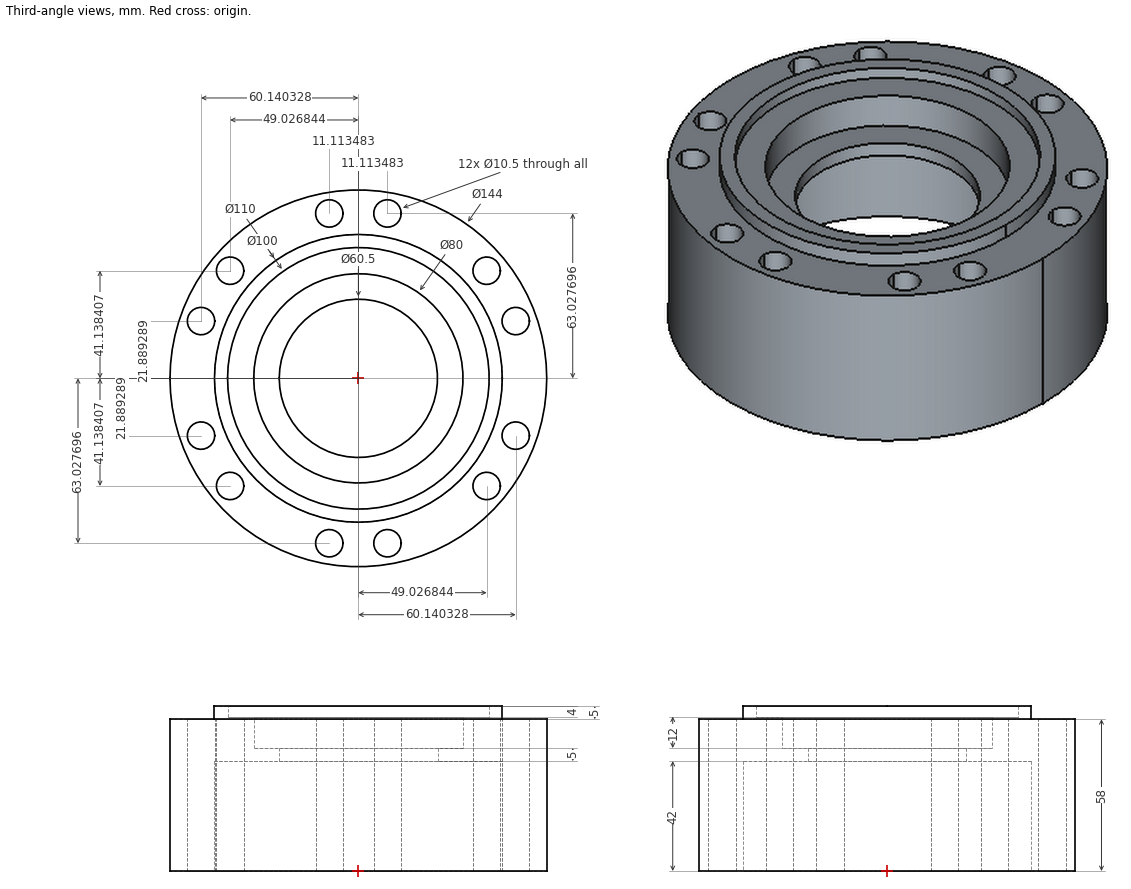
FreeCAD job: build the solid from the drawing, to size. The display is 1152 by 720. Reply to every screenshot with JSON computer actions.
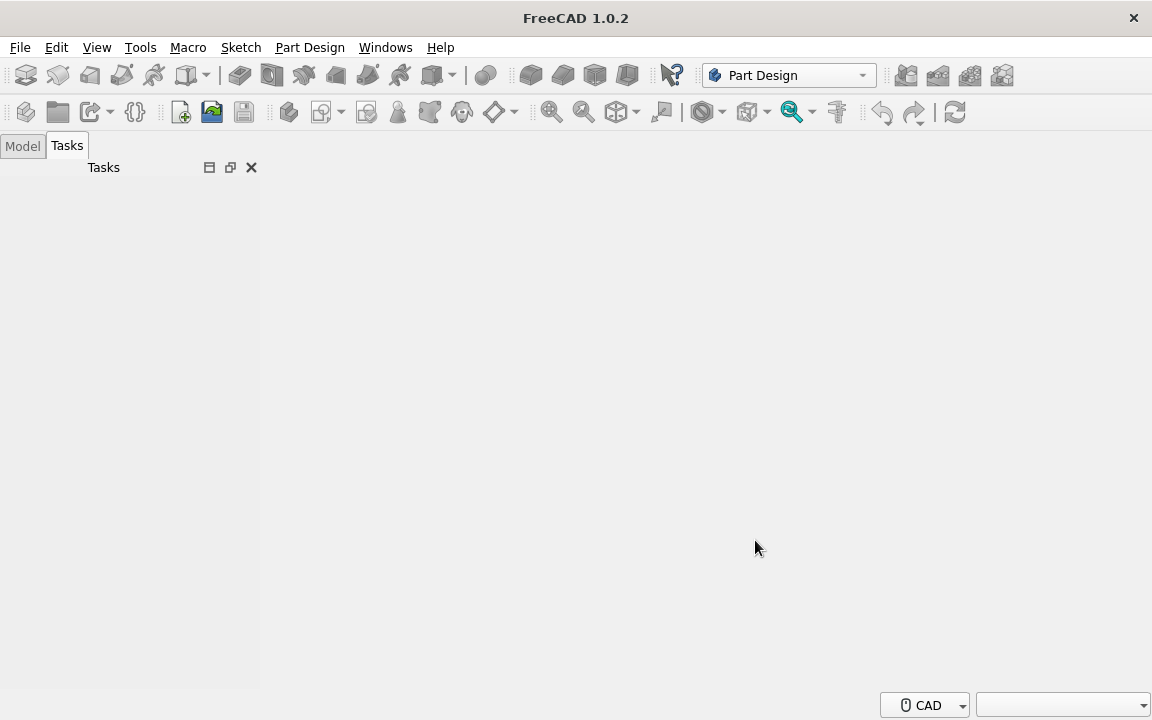
{"action": "left_click", "coordinate": [180, 112]}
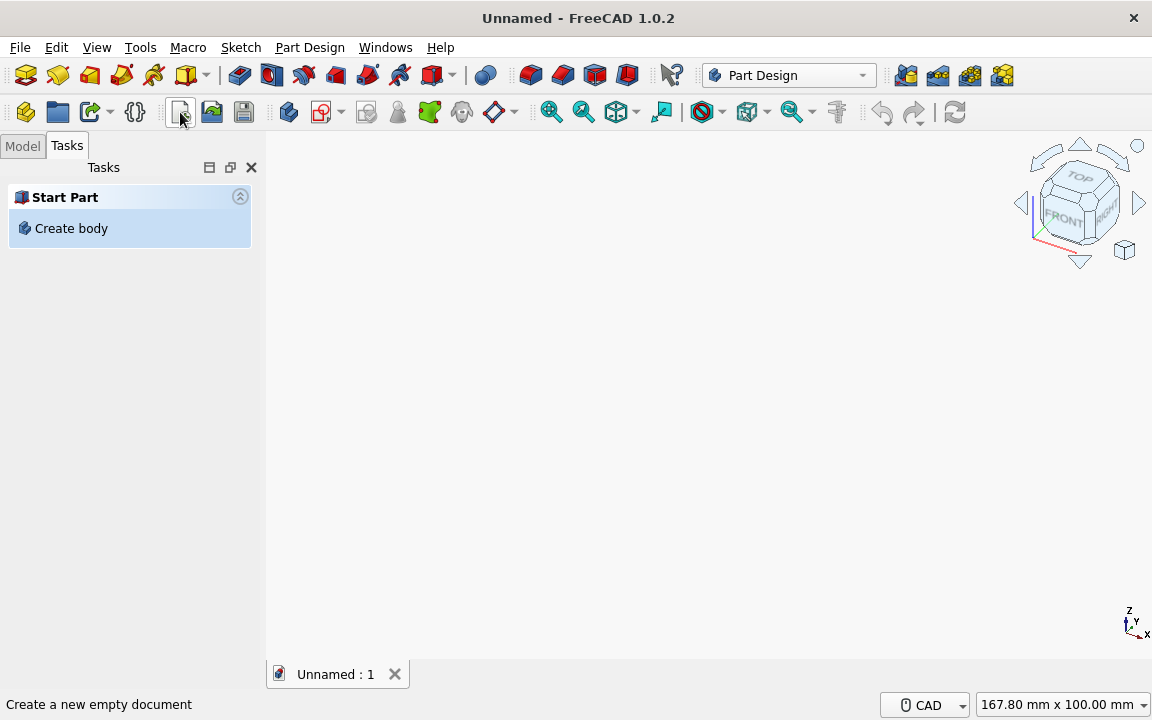
{"action": "left_click", "coordinate": [322, 112]}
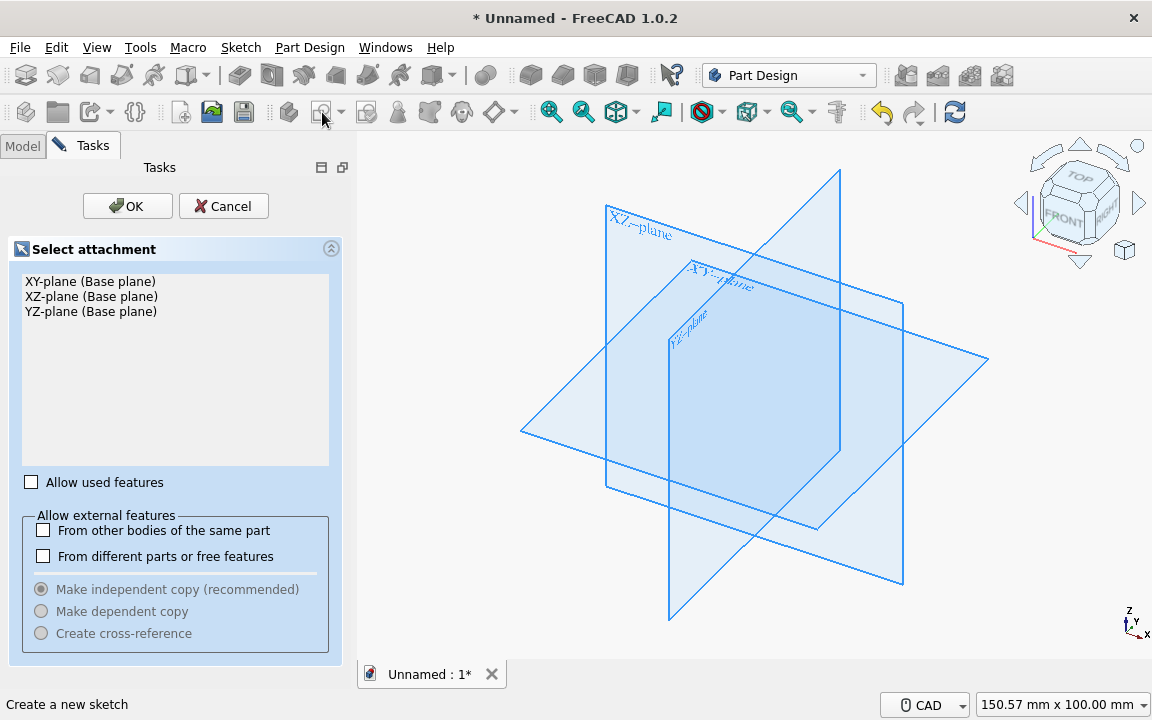
{"action": "left_click", "coordinate": [82, 282]}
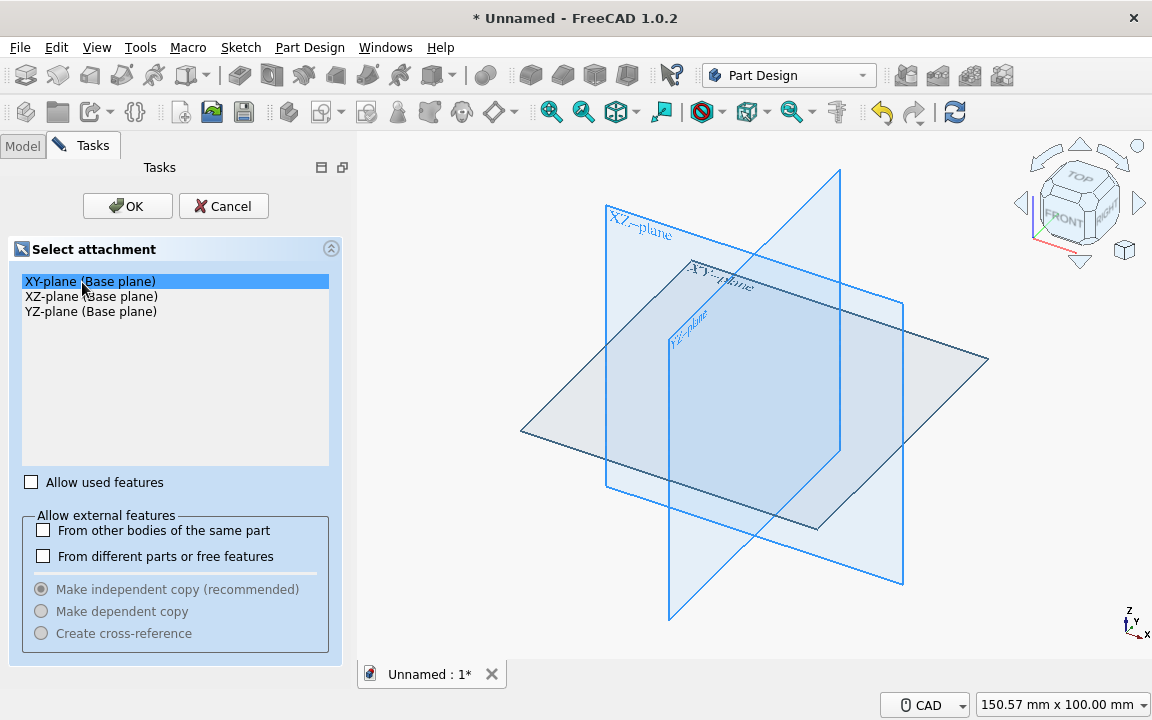
{"action": "left_click", "coordinate": [128, 206]}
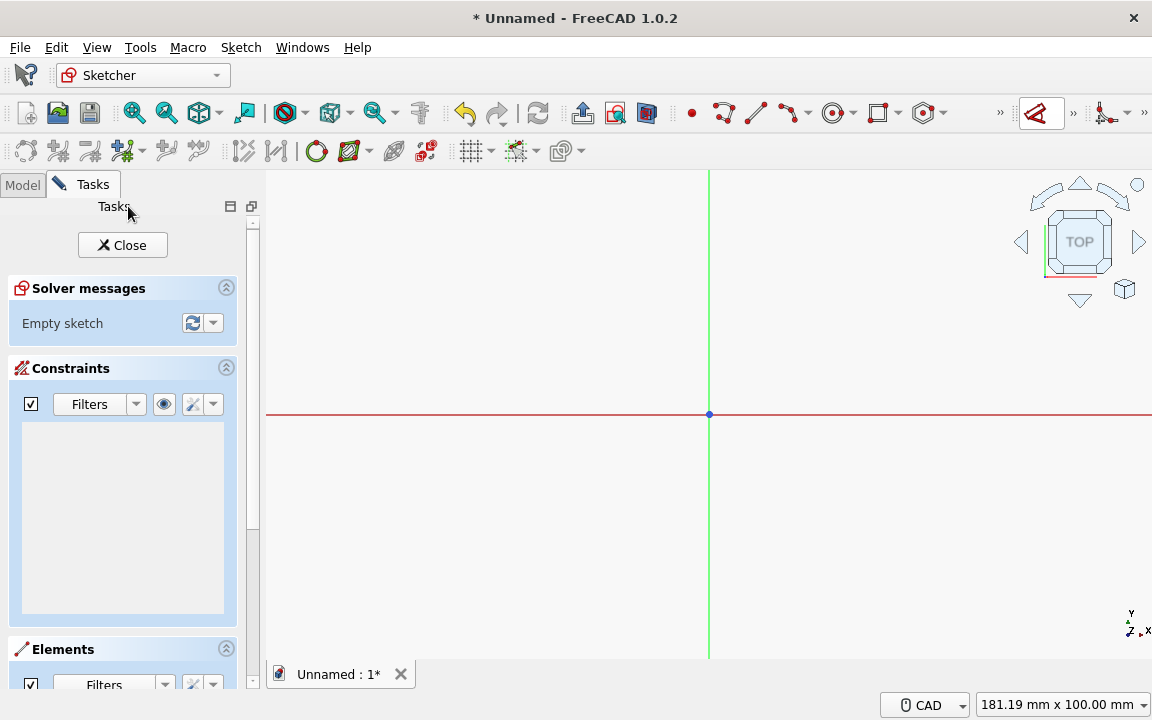
{"action": "scroll", "coordinate": [585, 414], "scroll_direction": "down", "scroll_amount": 4}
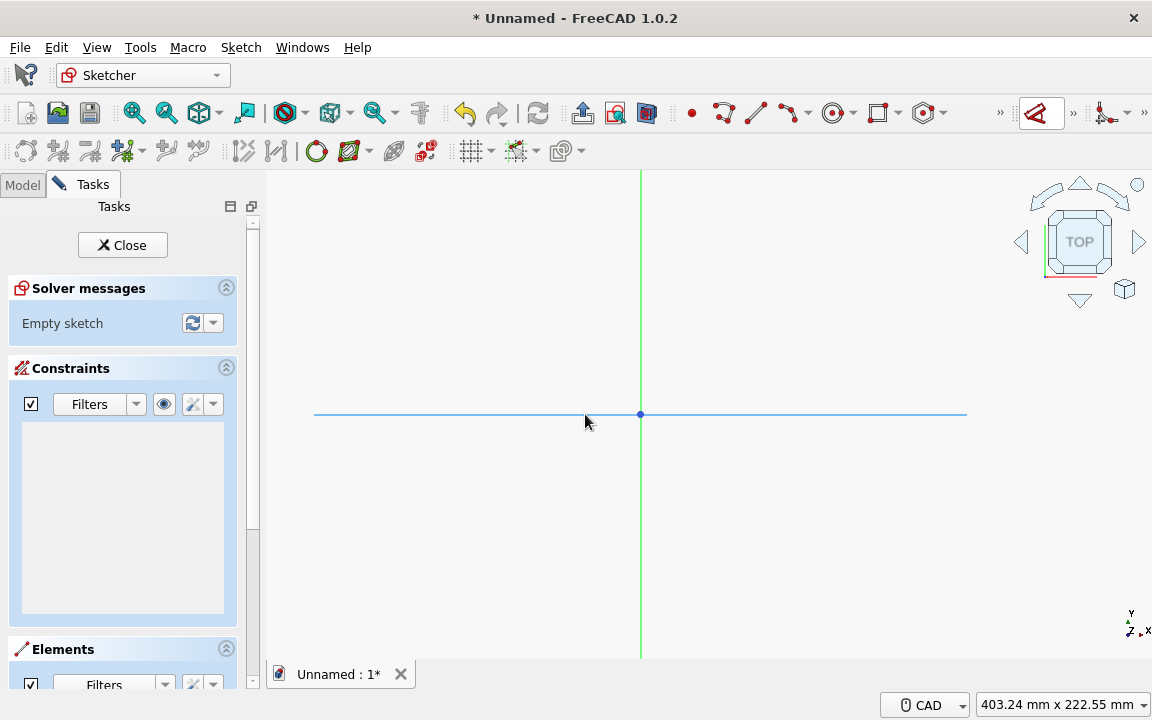
{"action": "left_click", "coordinate": [834, 114]}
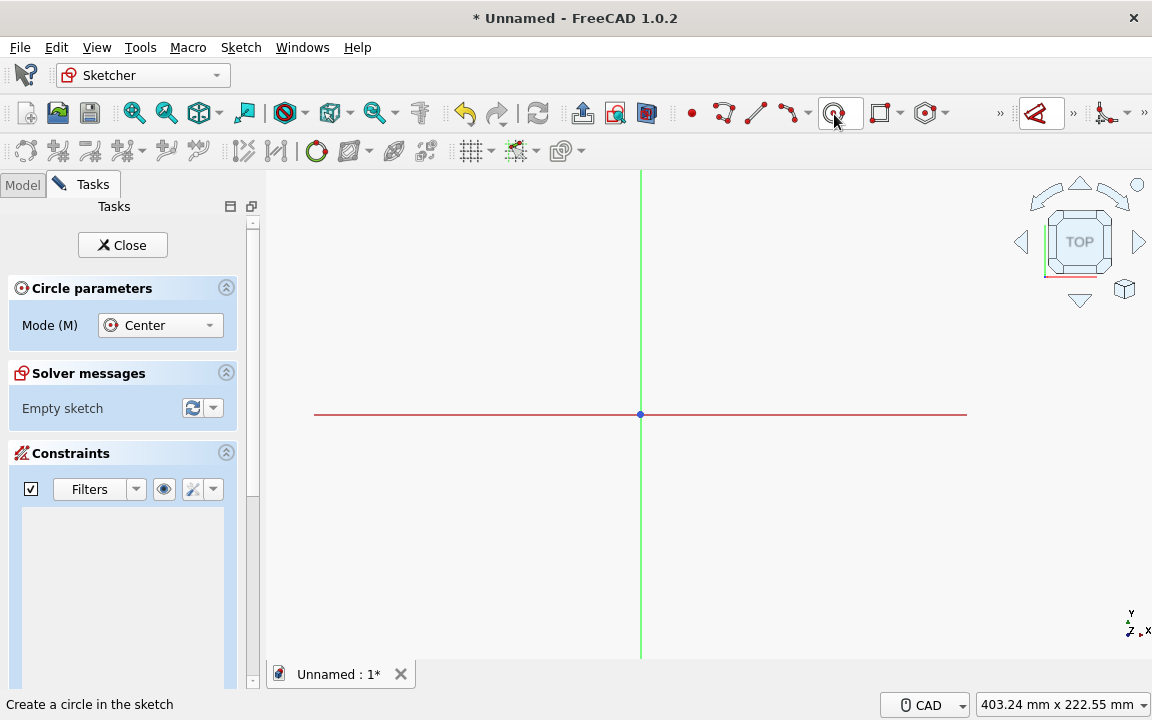
{"action": "left_click", "coordinate": [641, 414]}
{"action": "left_click", "coordinate": [753, 303]}
{"action": "key", "text": "Escape"}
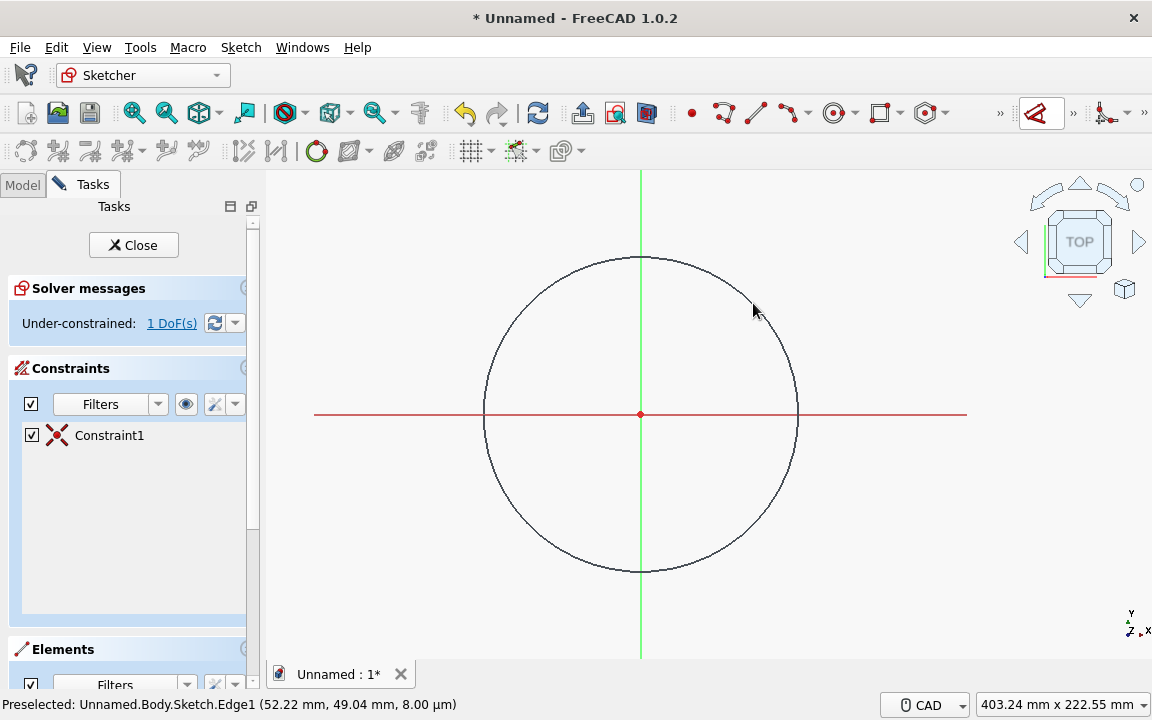
{"action": "key", "text": "d"}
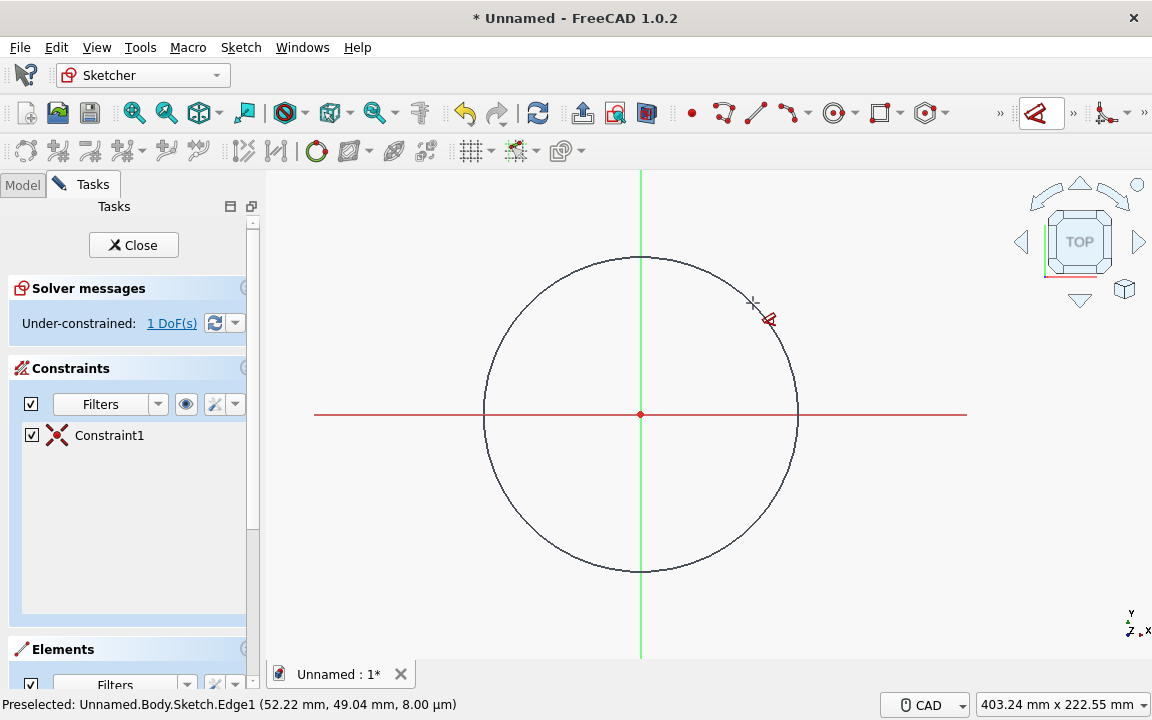
{"action": "left_click", "coordinate": [752, 303]}
{"action": "left_click", "coordinate": [775, 280]}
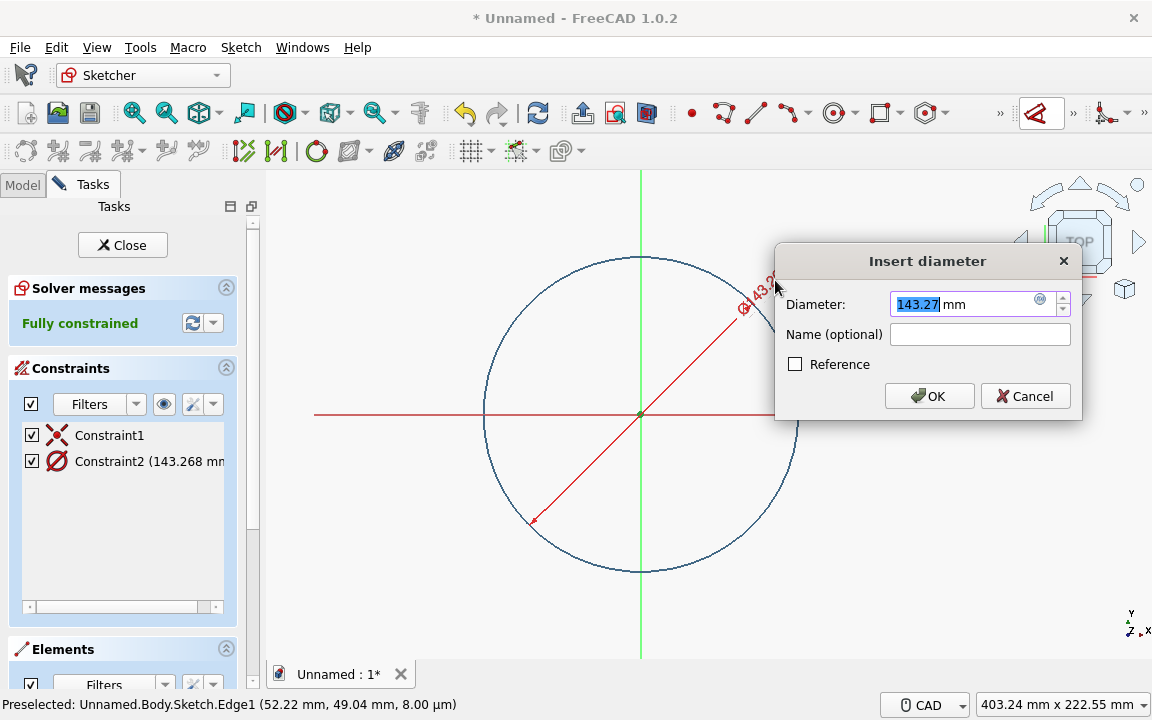
{"action": "type", "text": "144"}
{"action": "key", "text": "Return"}
{"action": "key", "text": "Escape"}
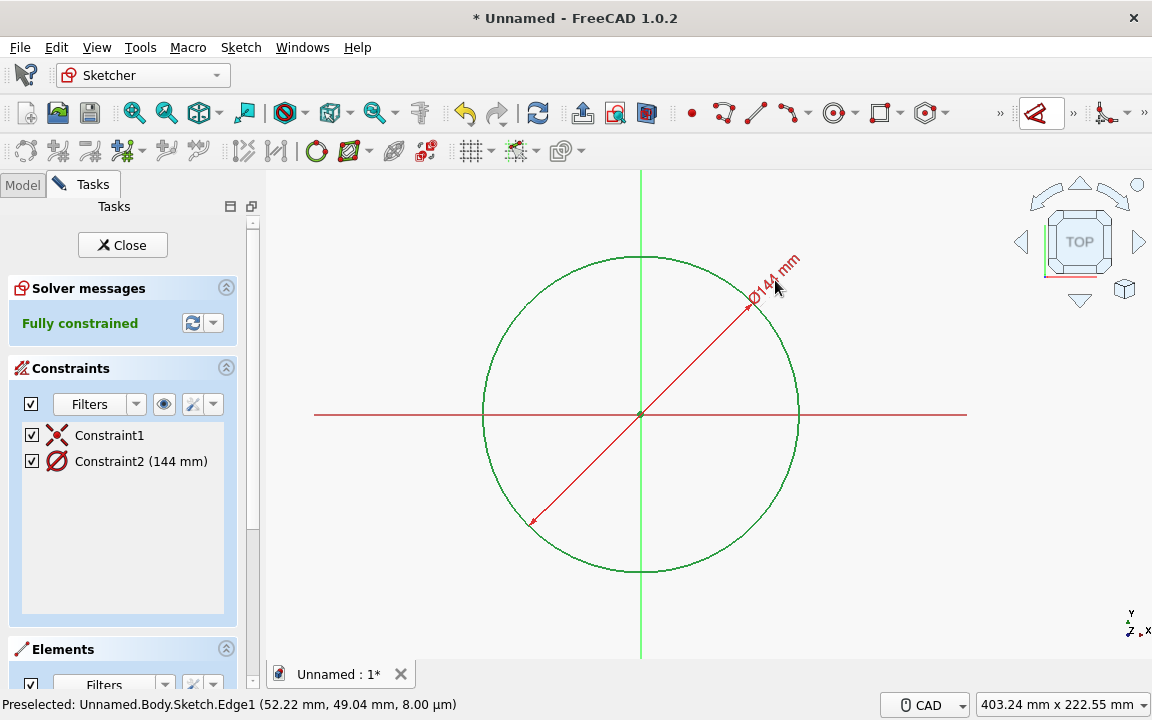
{"action": "left_click", "coordinate": [123, 245]}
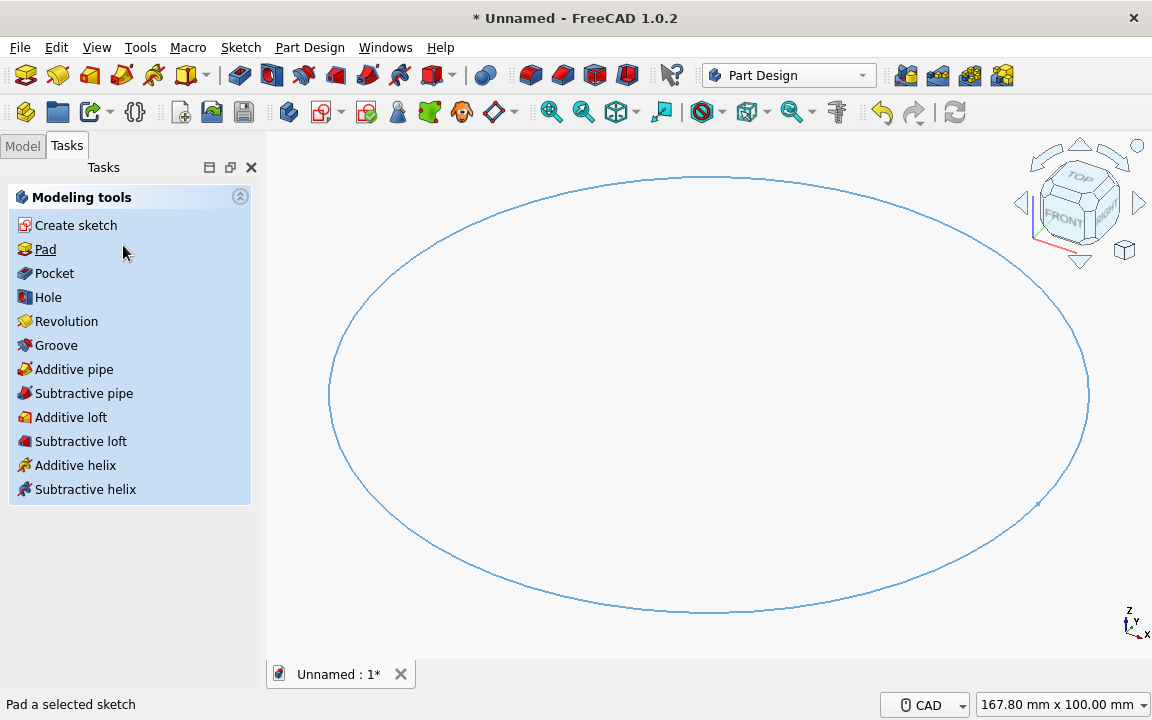
{"action": "left_click", "coordinate": [26, 76]}